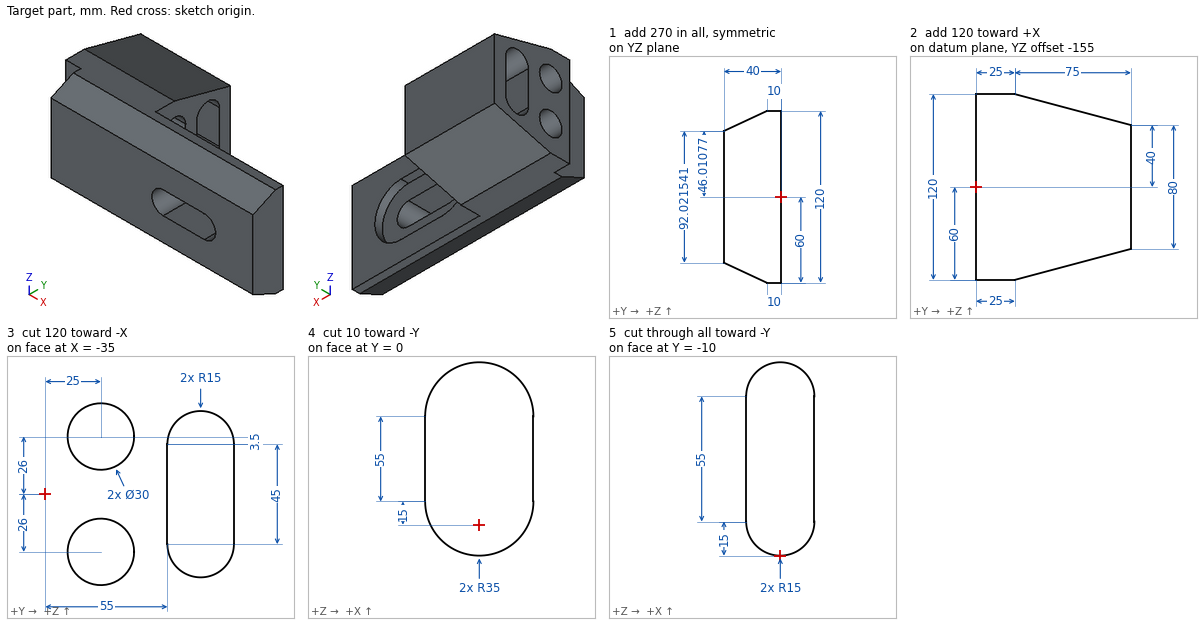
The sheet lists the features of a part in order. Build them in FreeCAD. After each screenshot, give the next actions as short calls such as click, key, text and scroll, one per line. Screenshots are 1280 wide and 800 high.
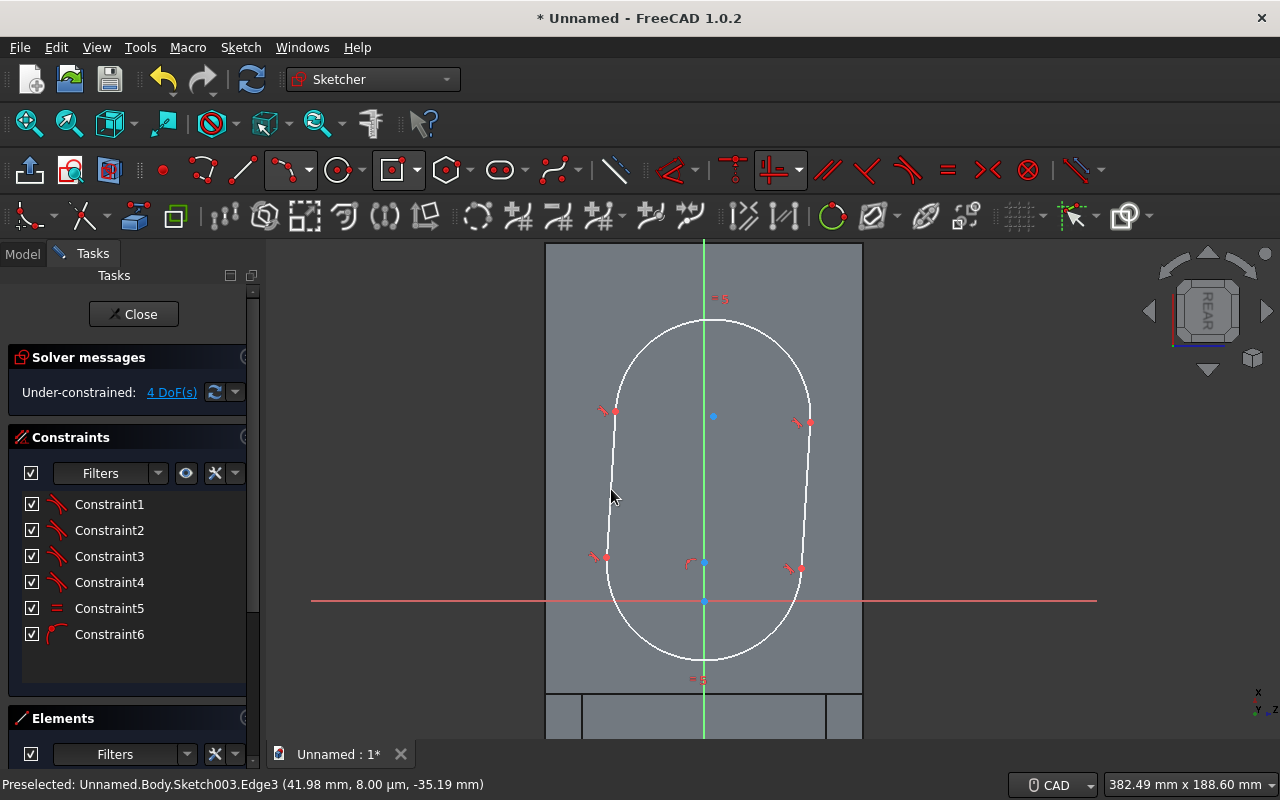
click(610, 513)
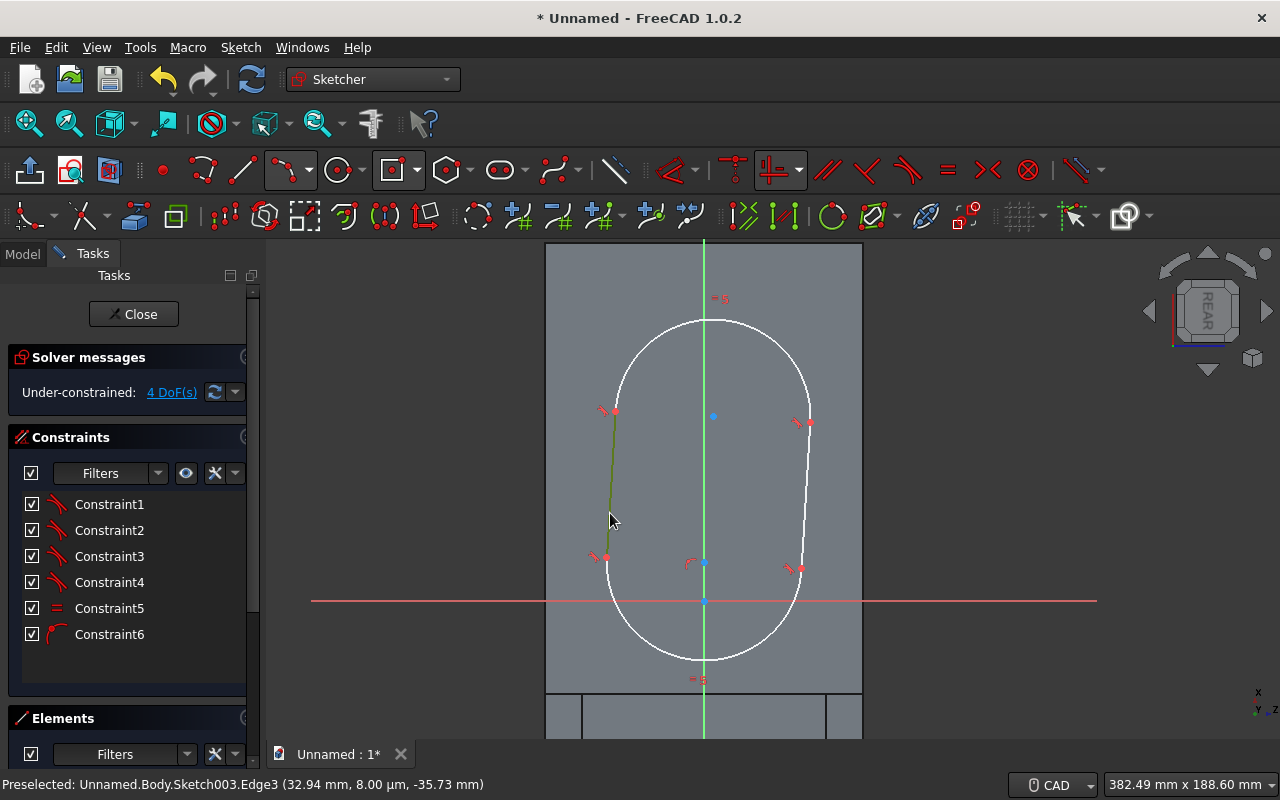
click(802, 170)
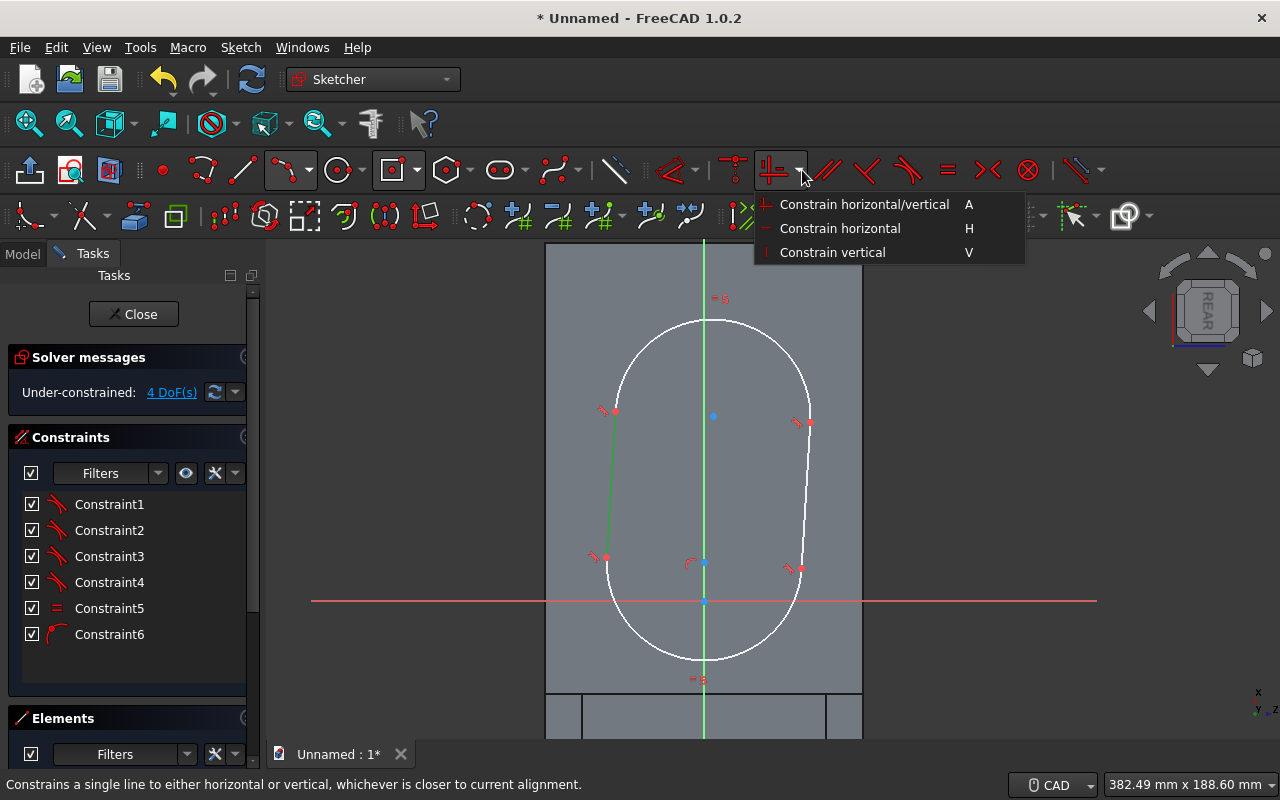
click(890, 252)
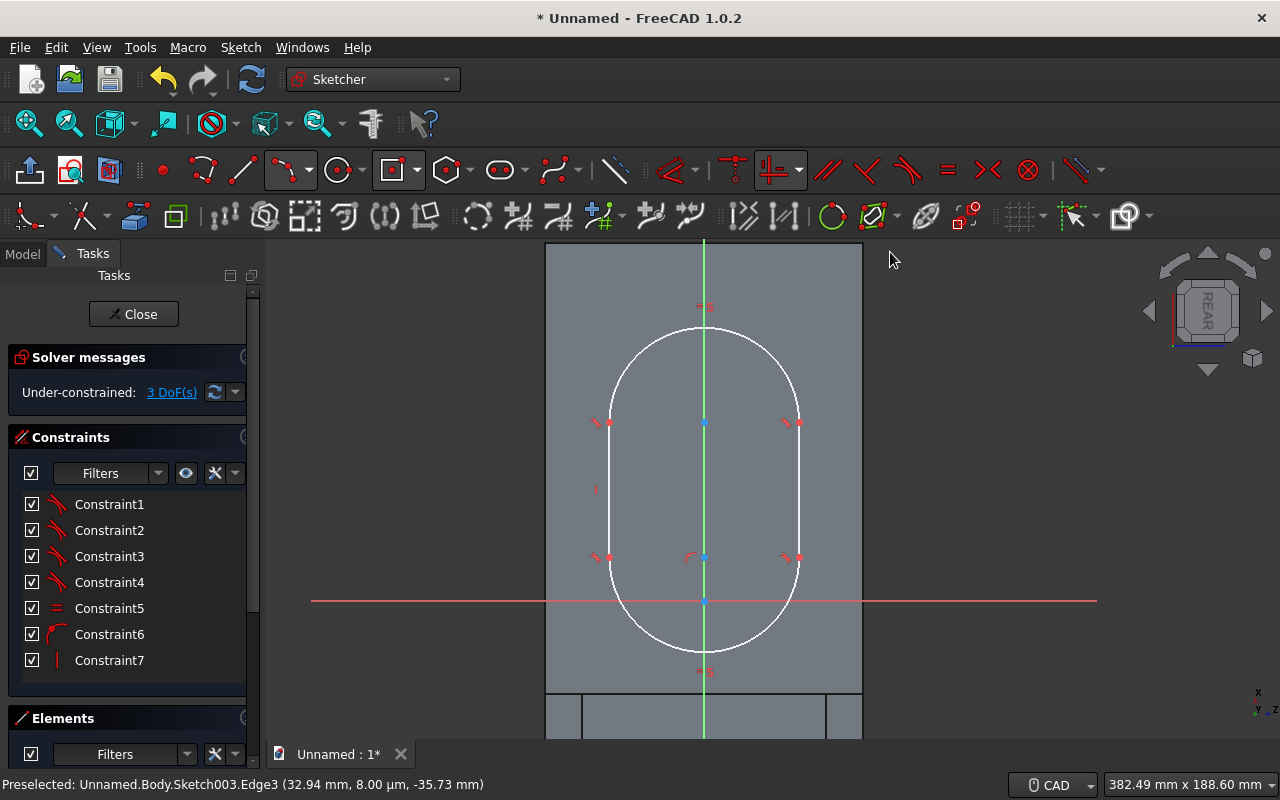
click(670, 170)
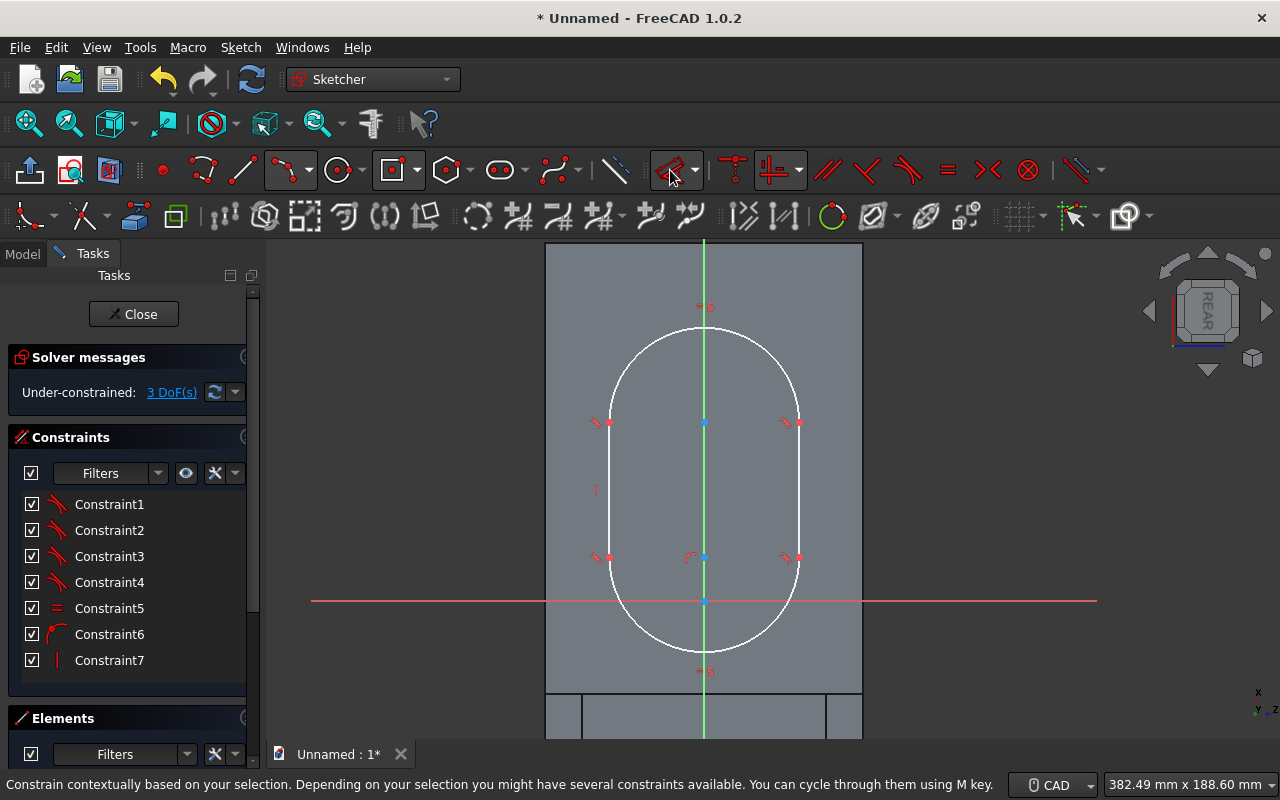
click(649, 634)
click(630, 660)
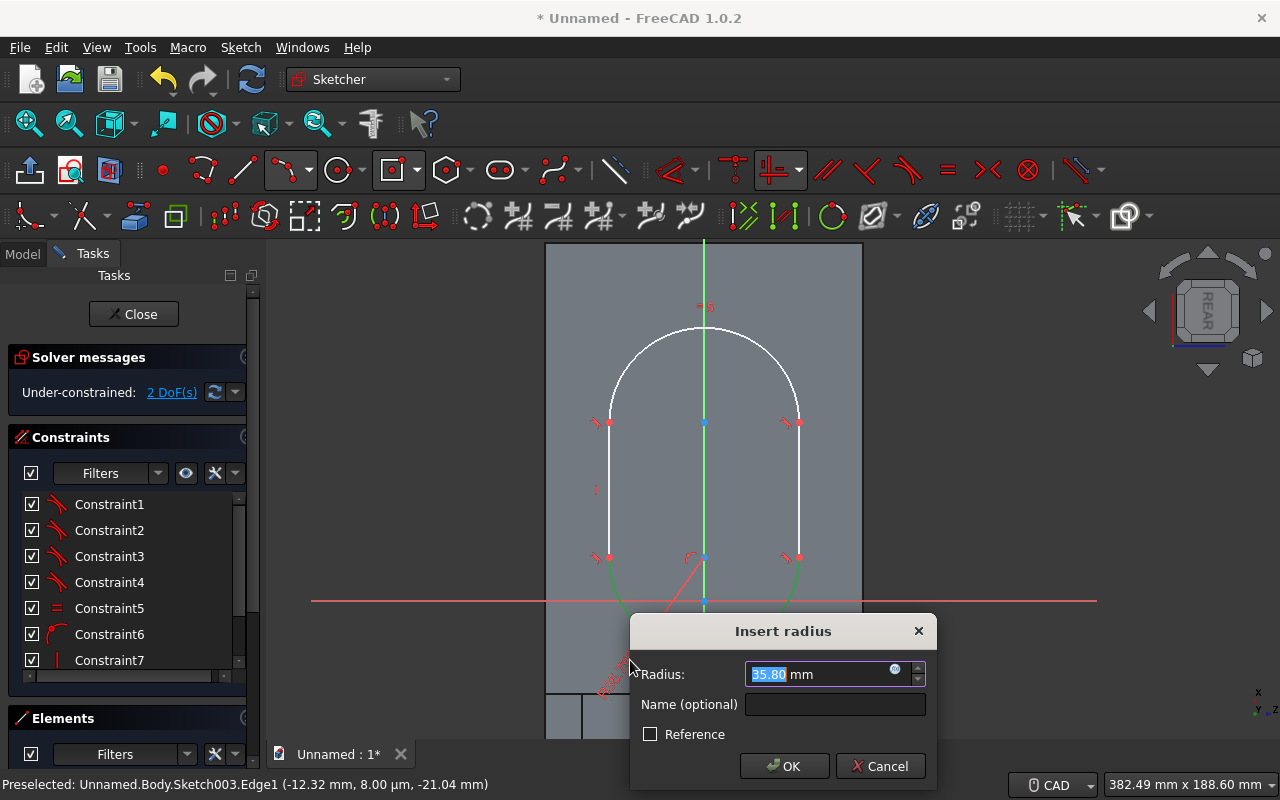
text(35)
key(Return)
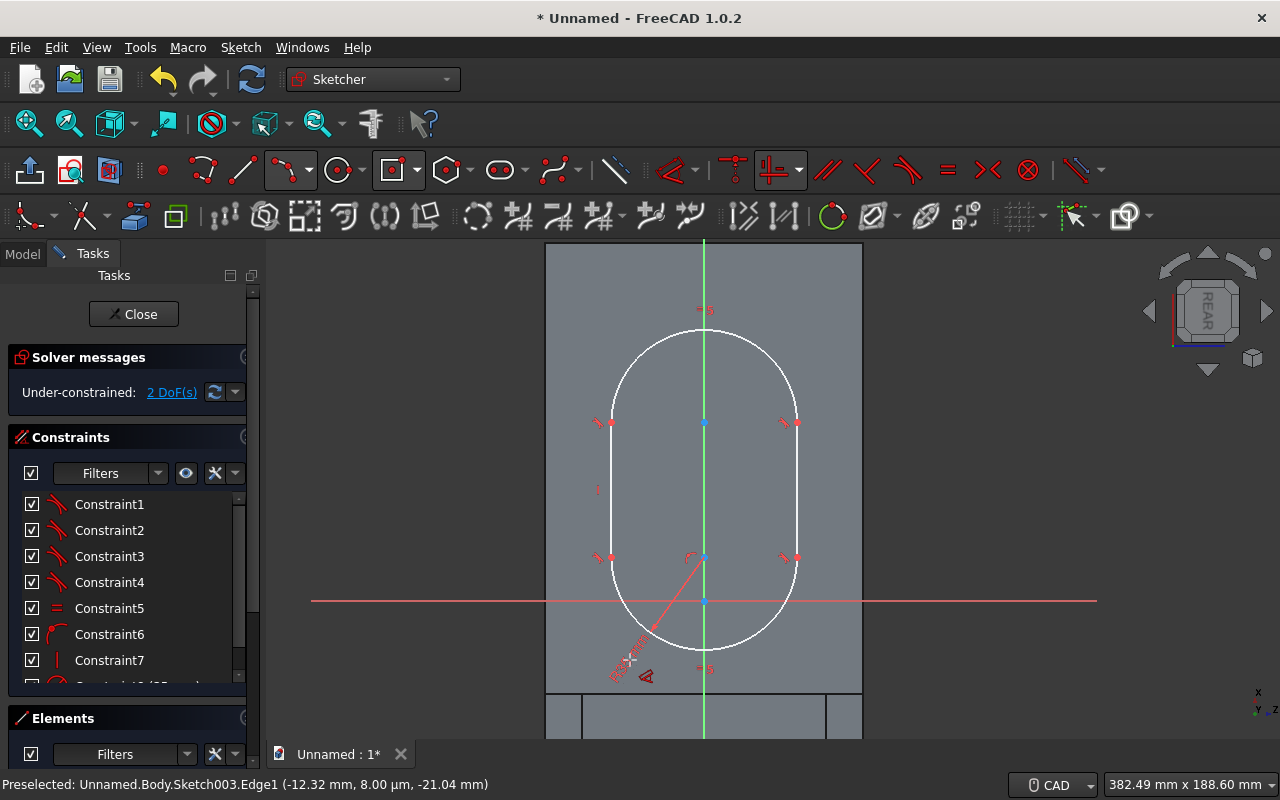
click(611, 517)
click(577, 490)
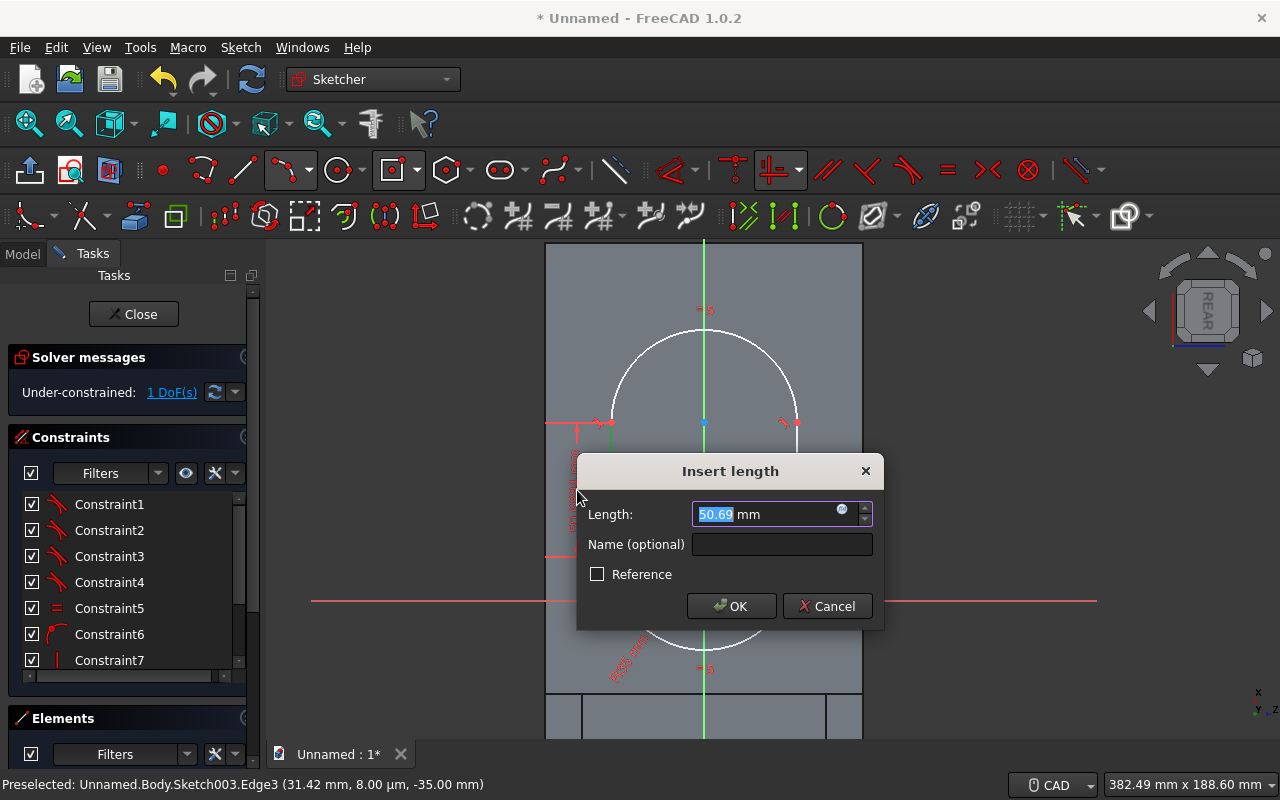
text(55)
key(Return)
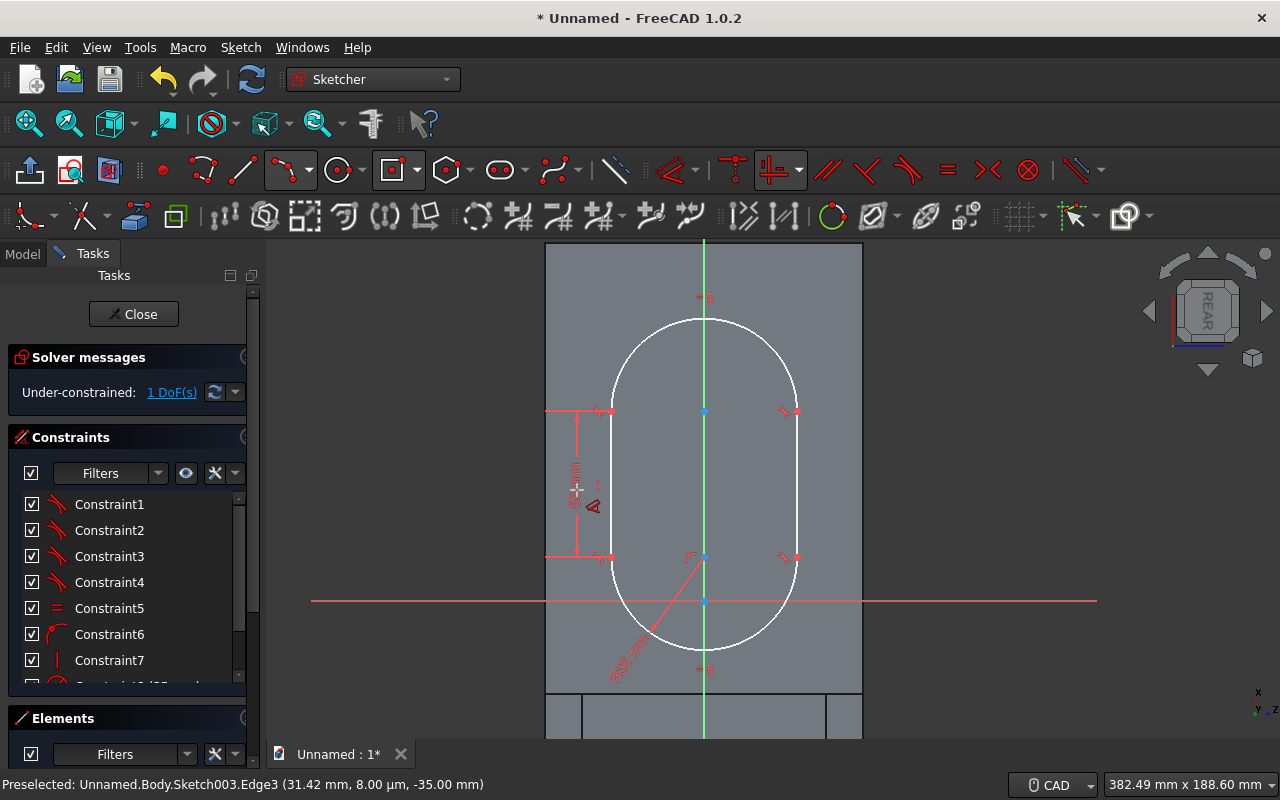
click(611, 557)
click(577, 579)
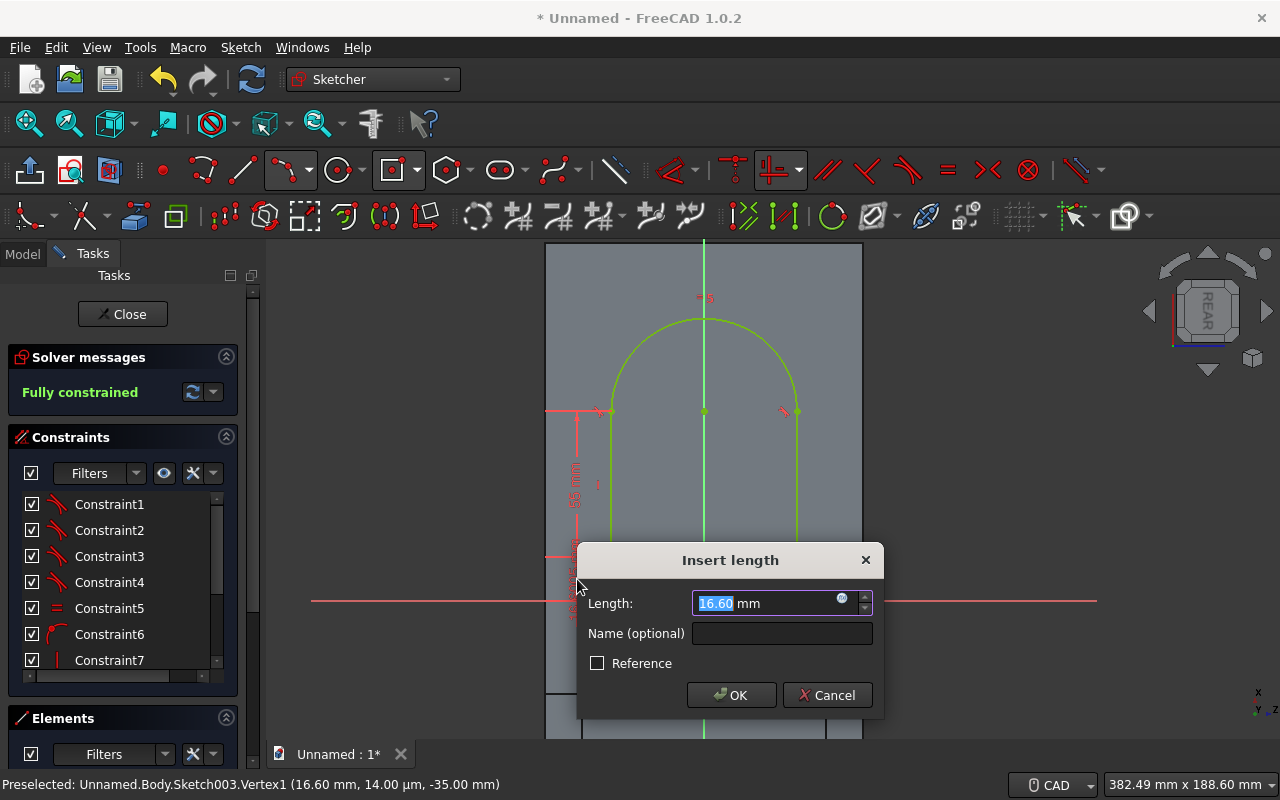
text(15)
key(Return)
key(Escape)